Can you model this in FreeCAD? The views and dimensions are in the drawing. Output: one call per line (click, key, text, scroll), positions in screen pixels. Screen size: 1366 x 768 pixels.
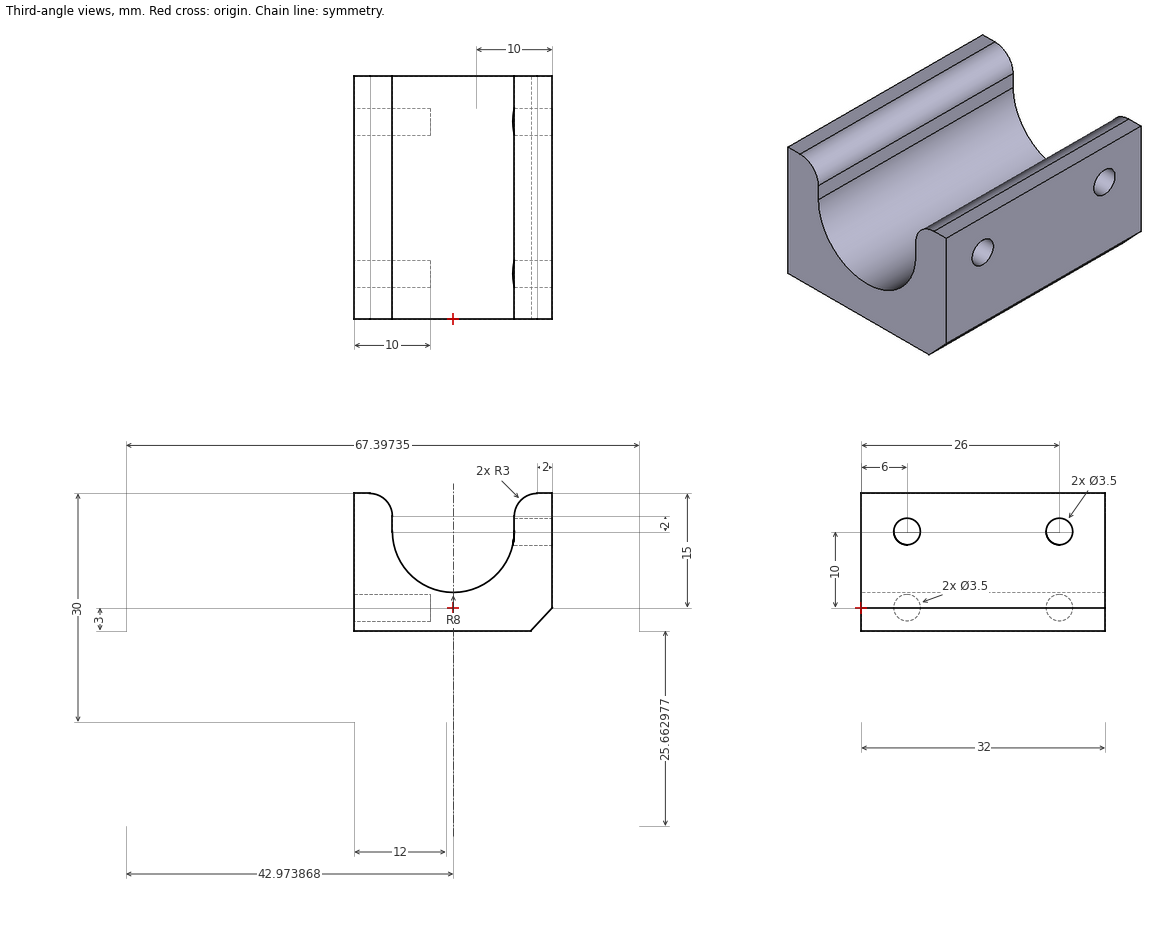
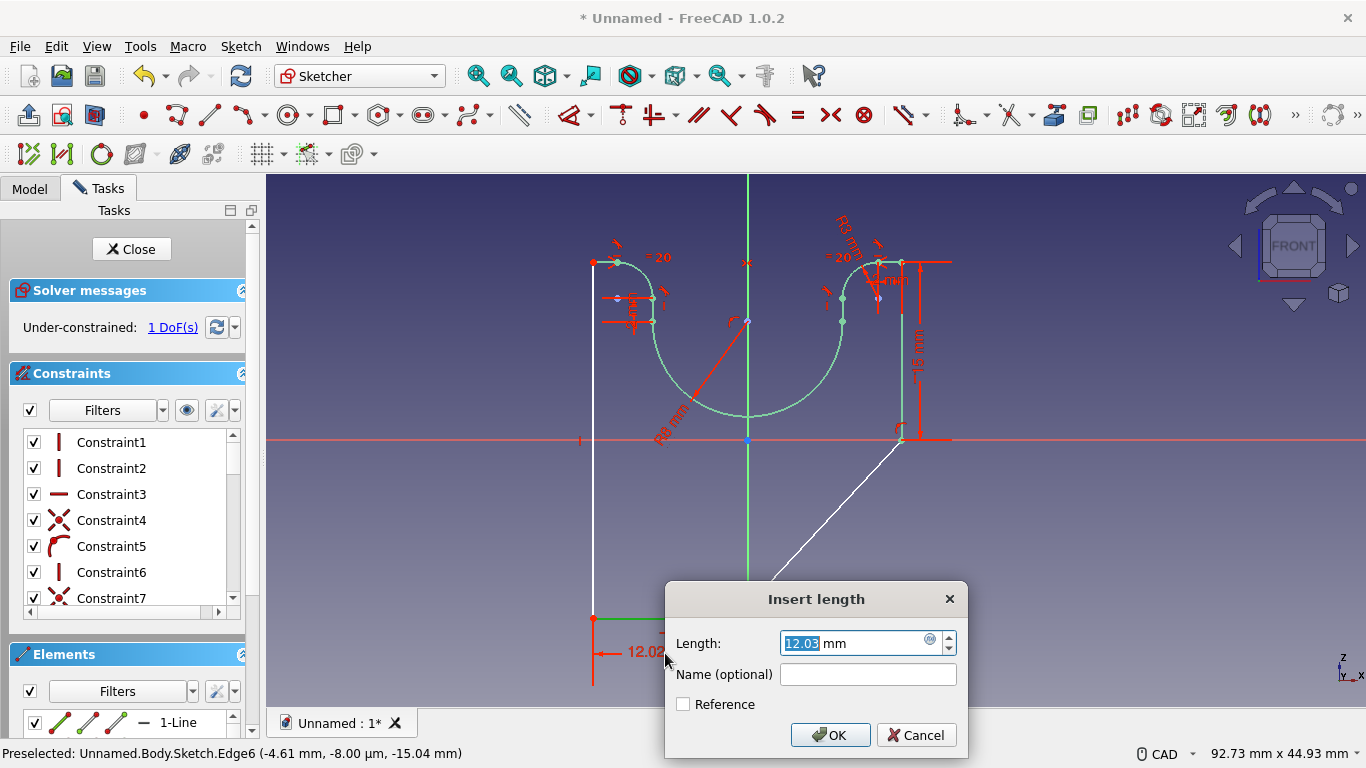
text(12)
key(Return)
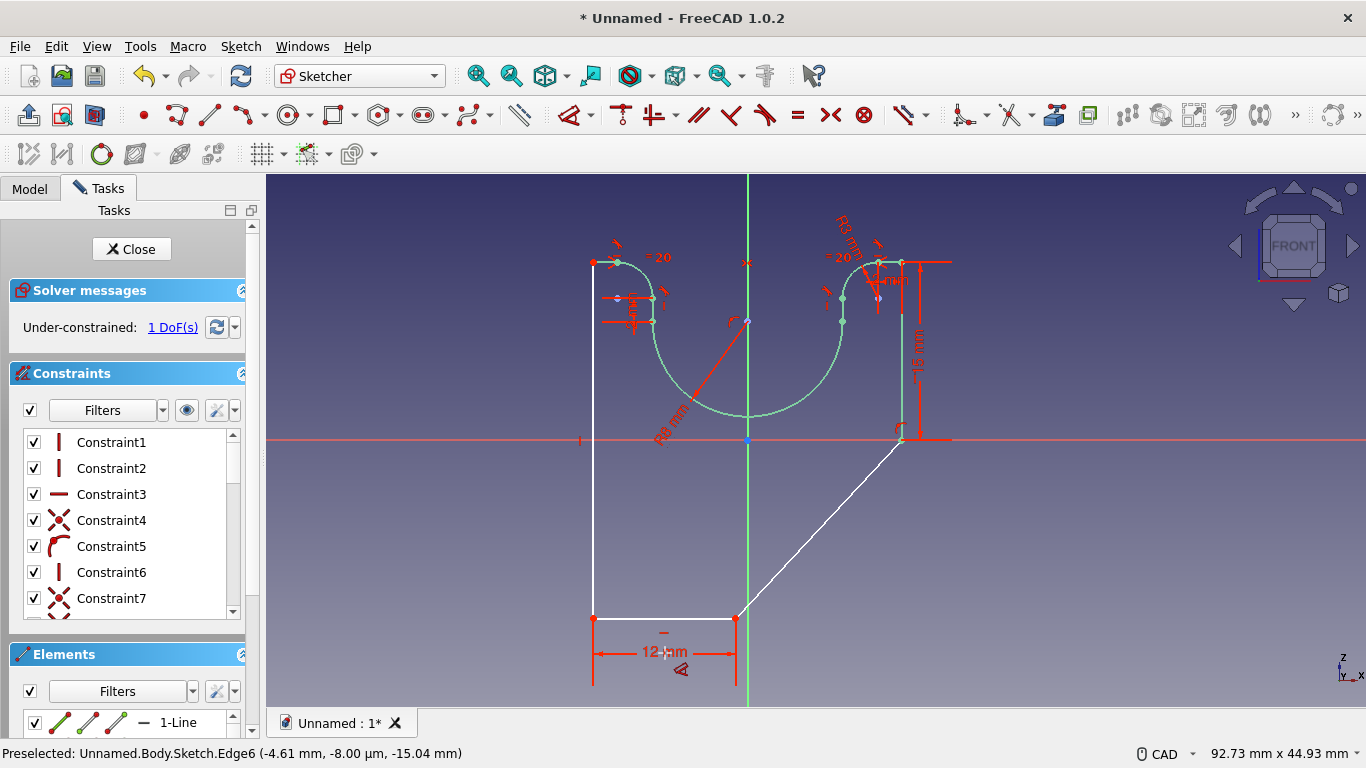
click(593, 512)
click(559, 359)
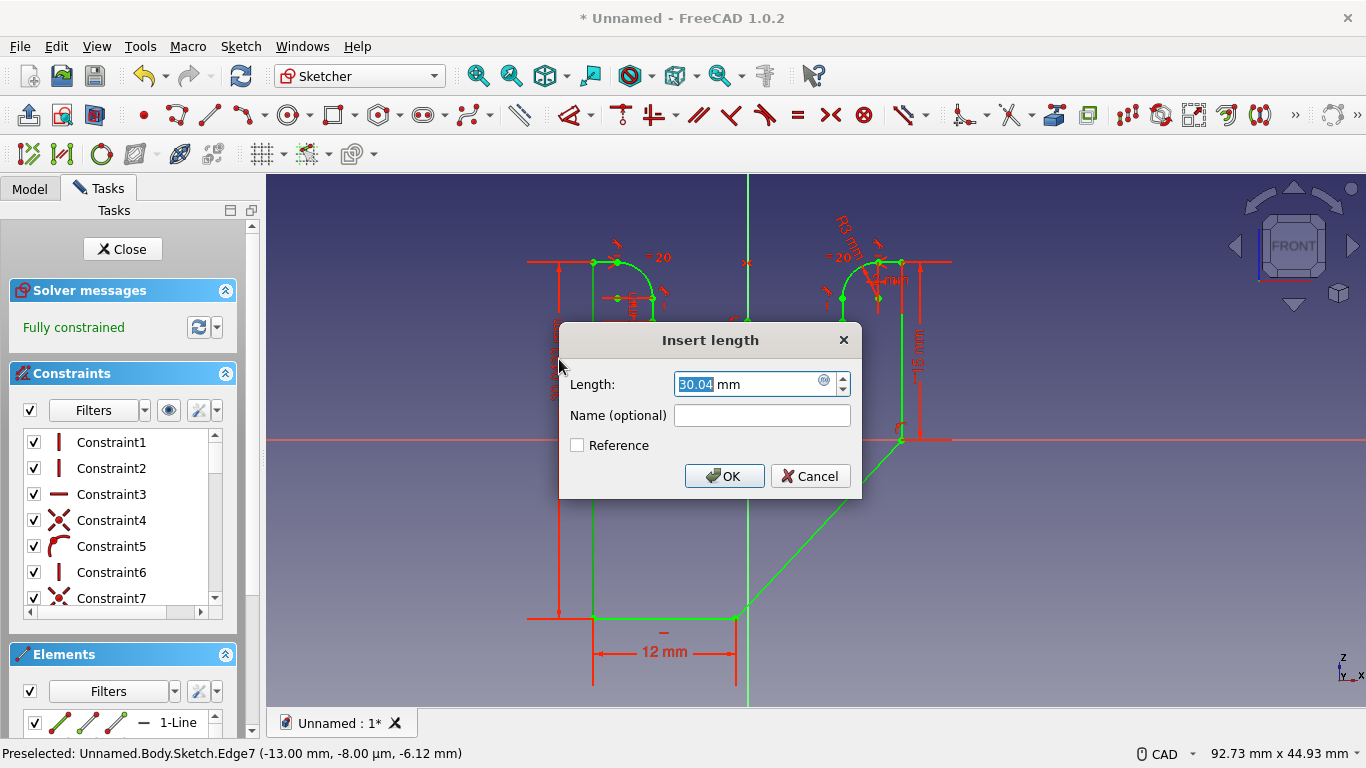
text(30)
key(Return)
key(Escape)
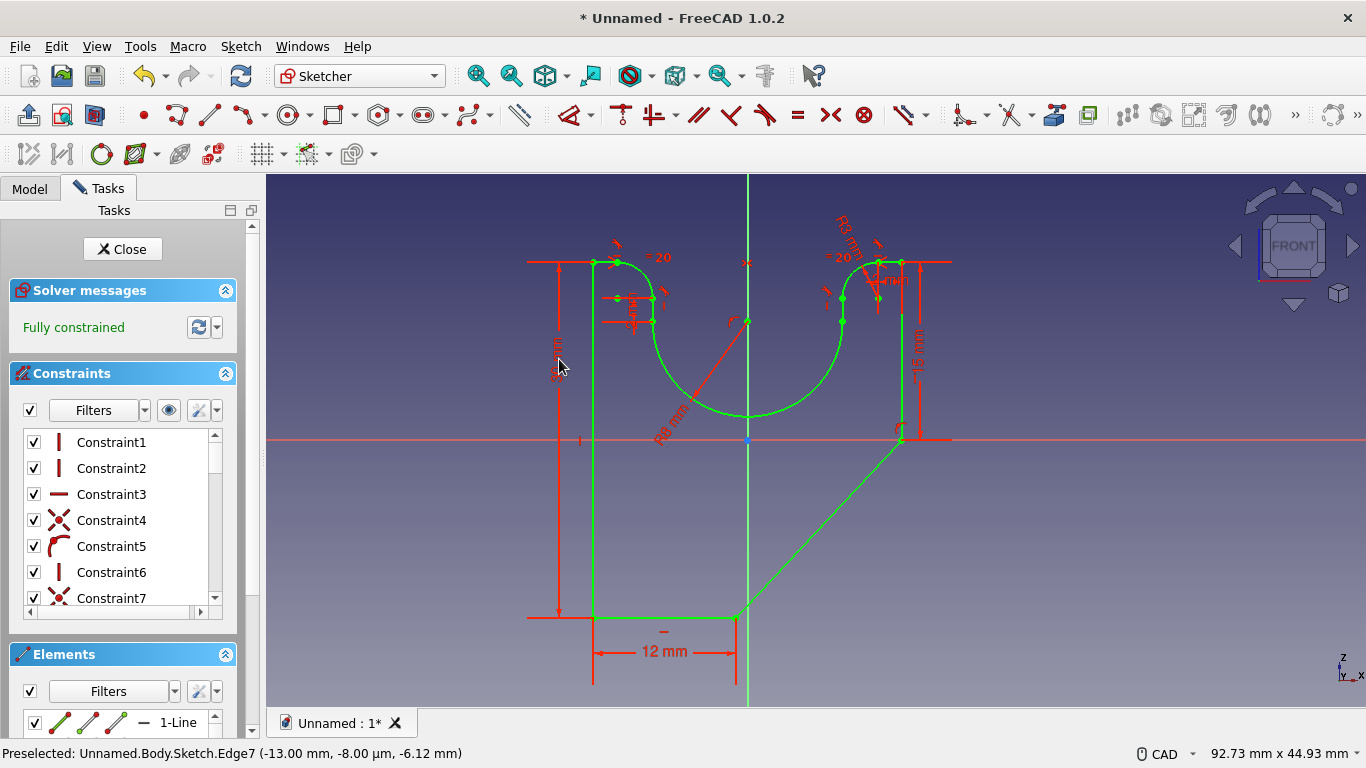
click(123, 249)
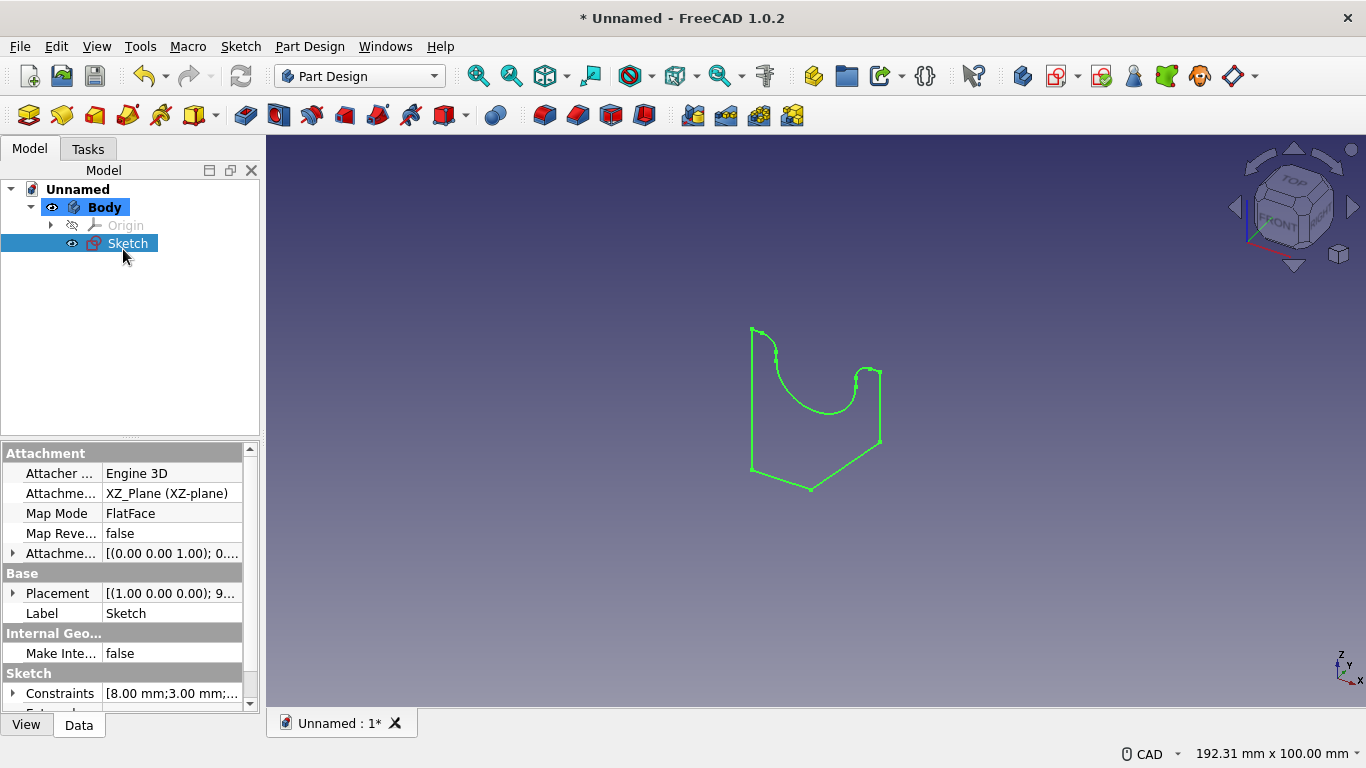
click(29, 116)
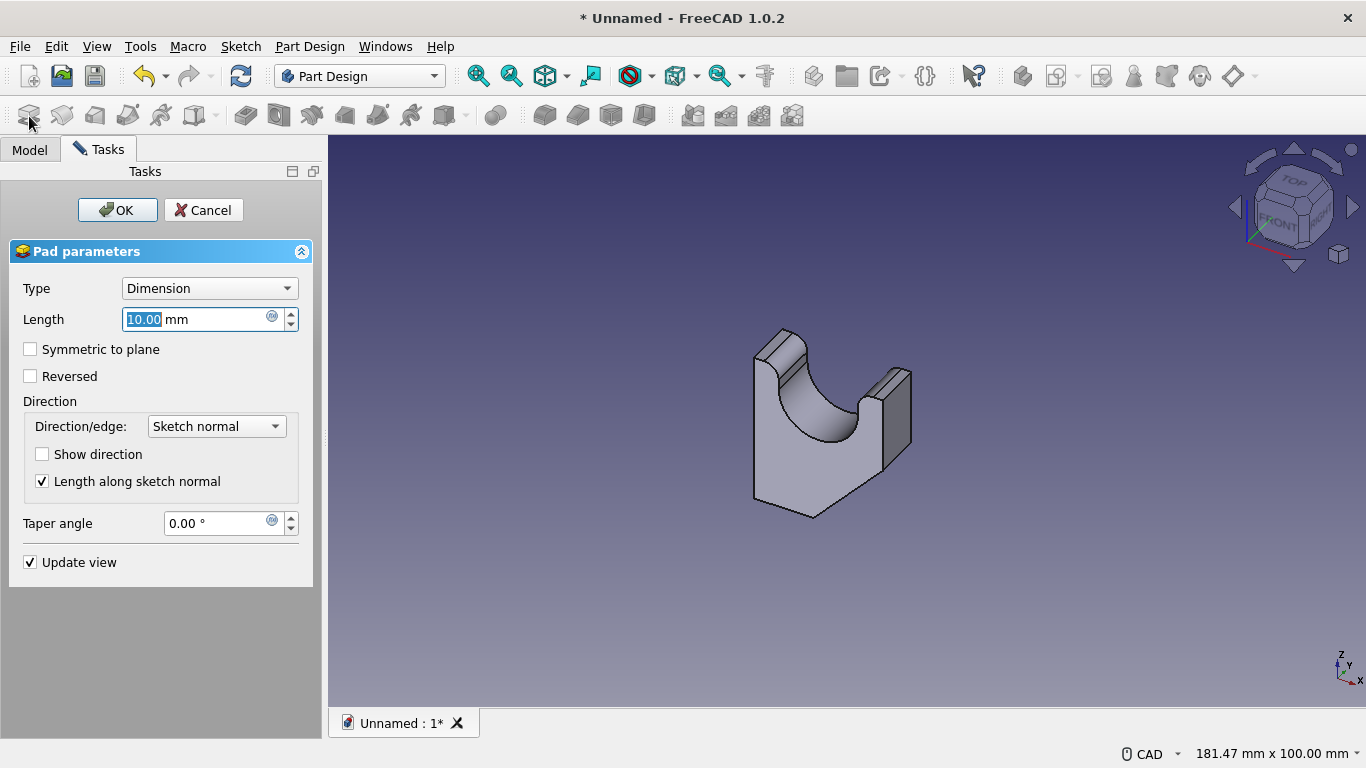
text(32)
key(Tab)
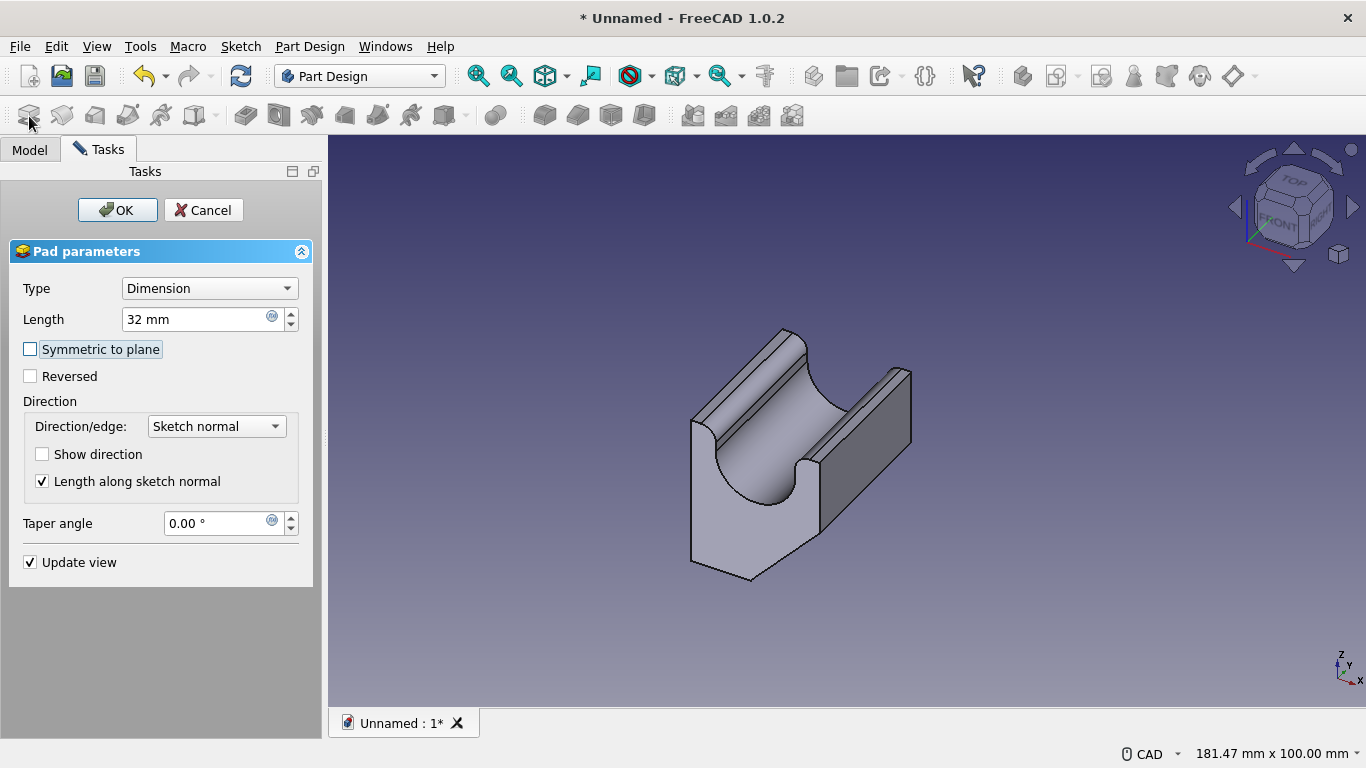
click(31, 376)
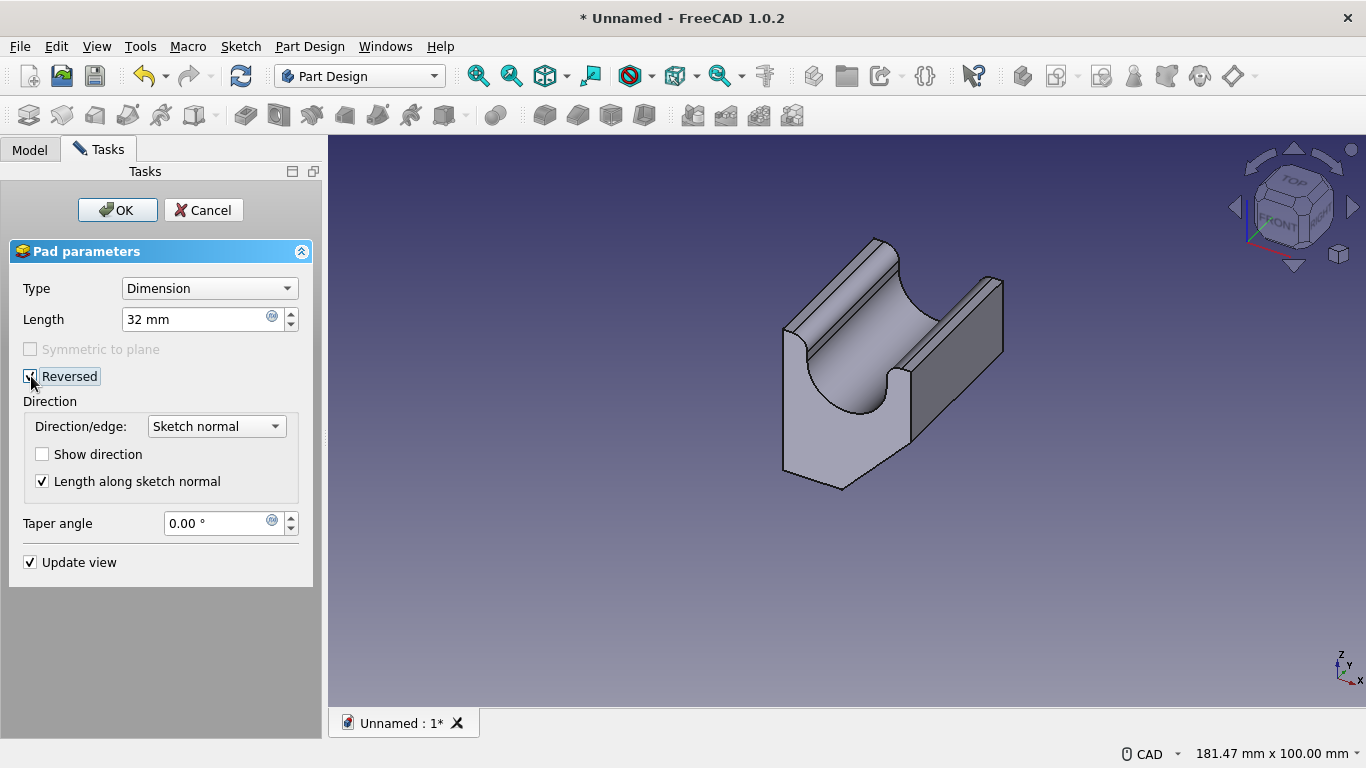
click(118, 210)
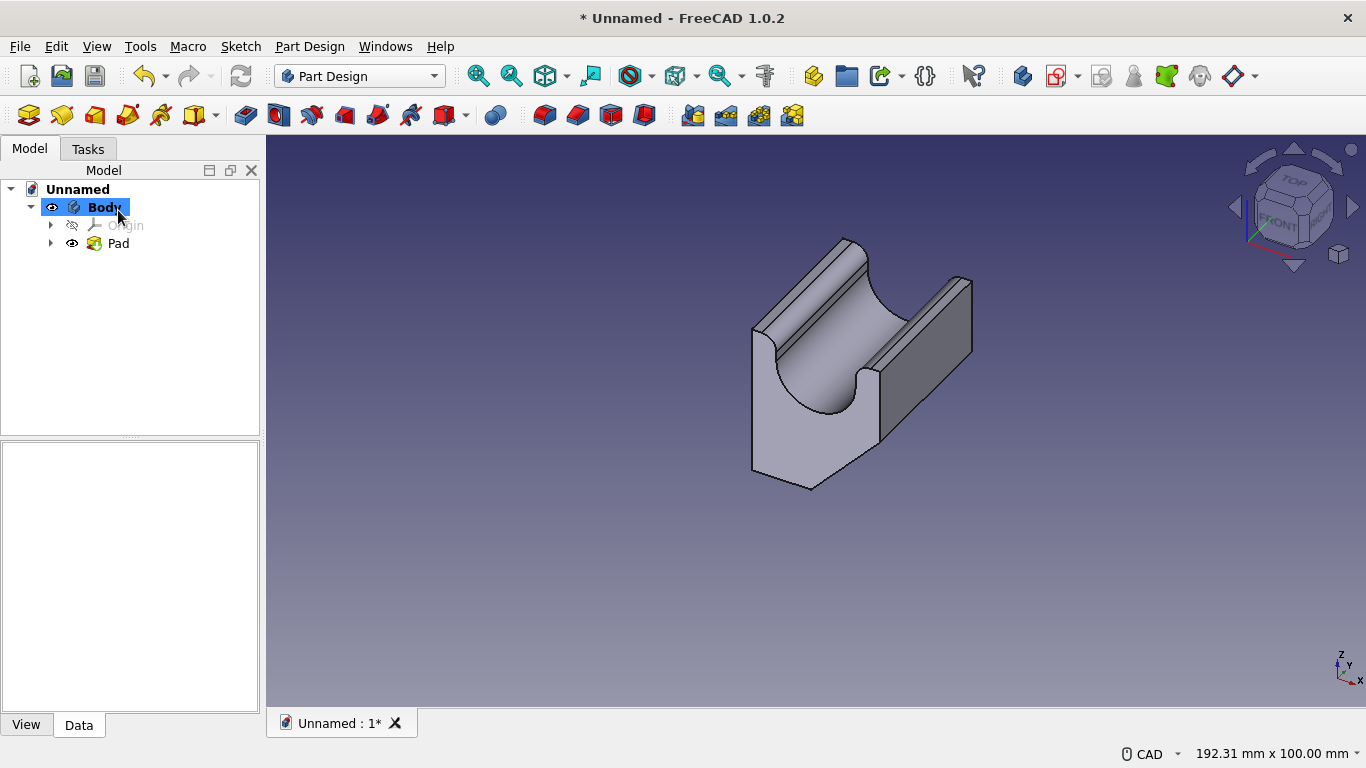
click(926, 361)